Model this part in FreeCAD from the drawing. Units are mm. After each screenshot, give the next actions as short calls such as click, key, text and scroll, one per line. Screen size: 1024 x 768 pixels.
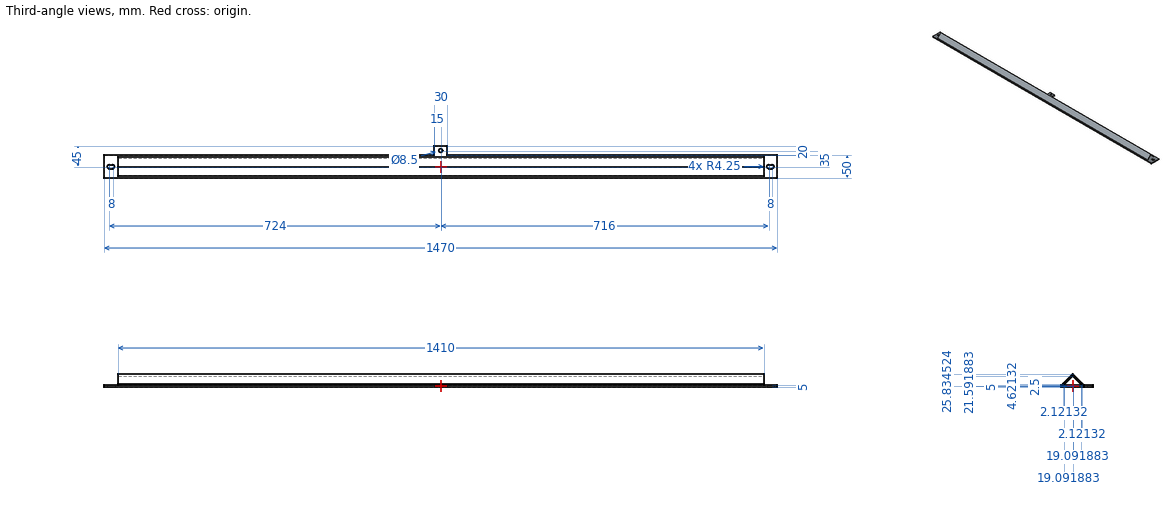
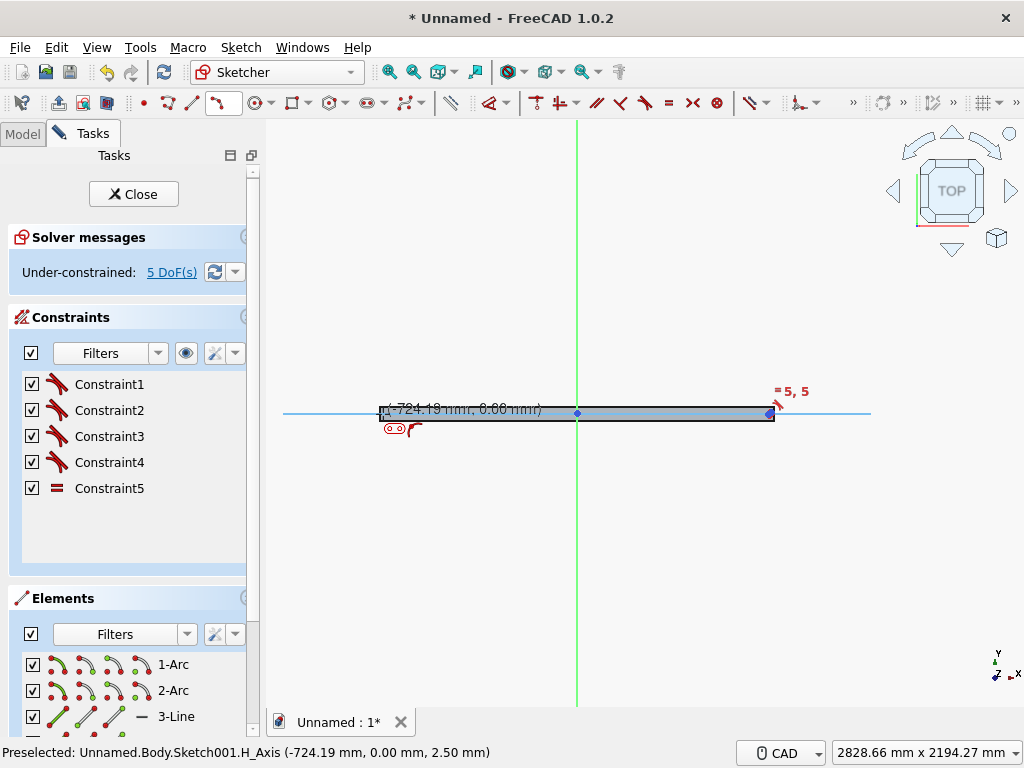
click(383, 414)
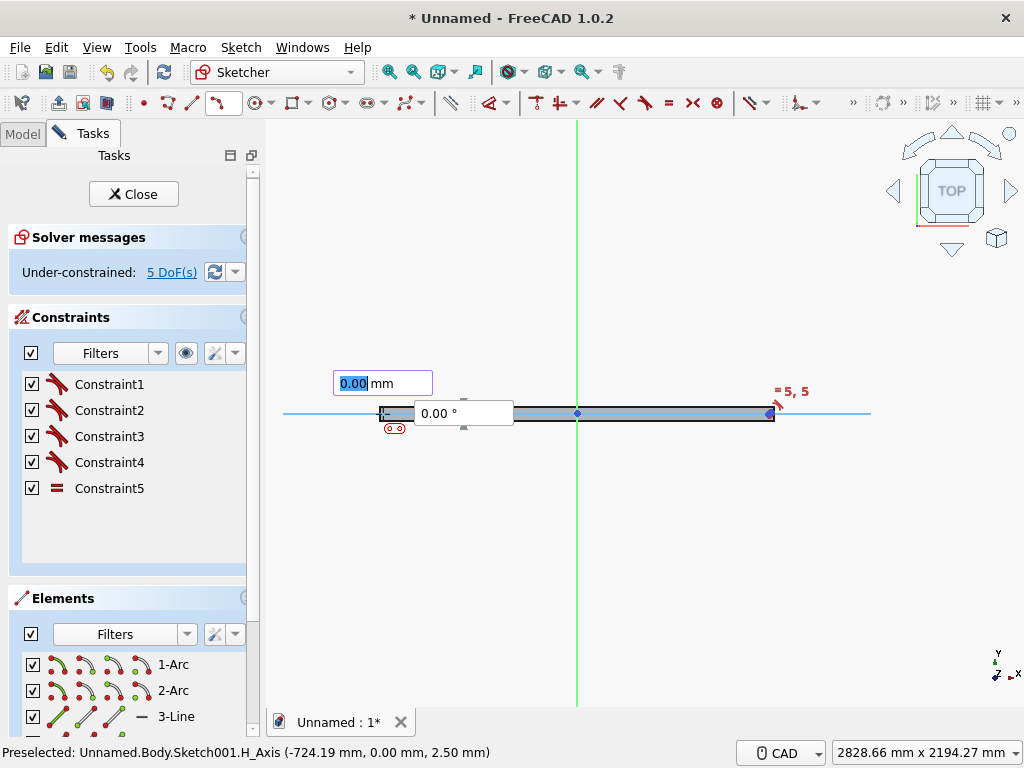
scroll(385, 414, up, 11)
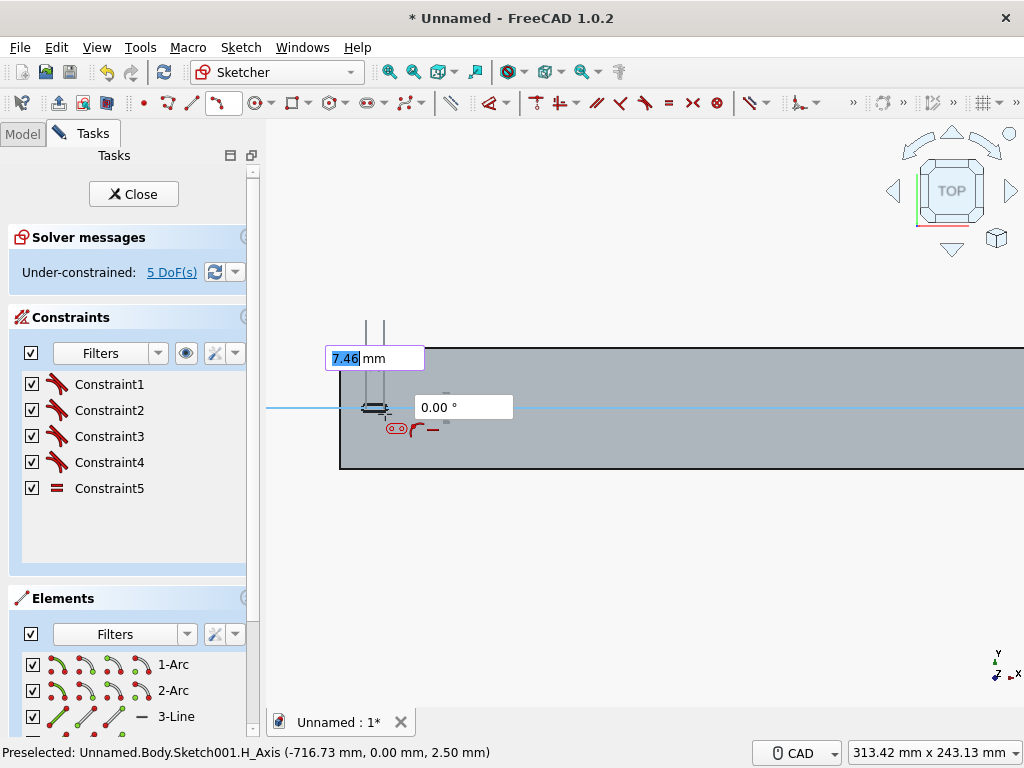
click(386, 399)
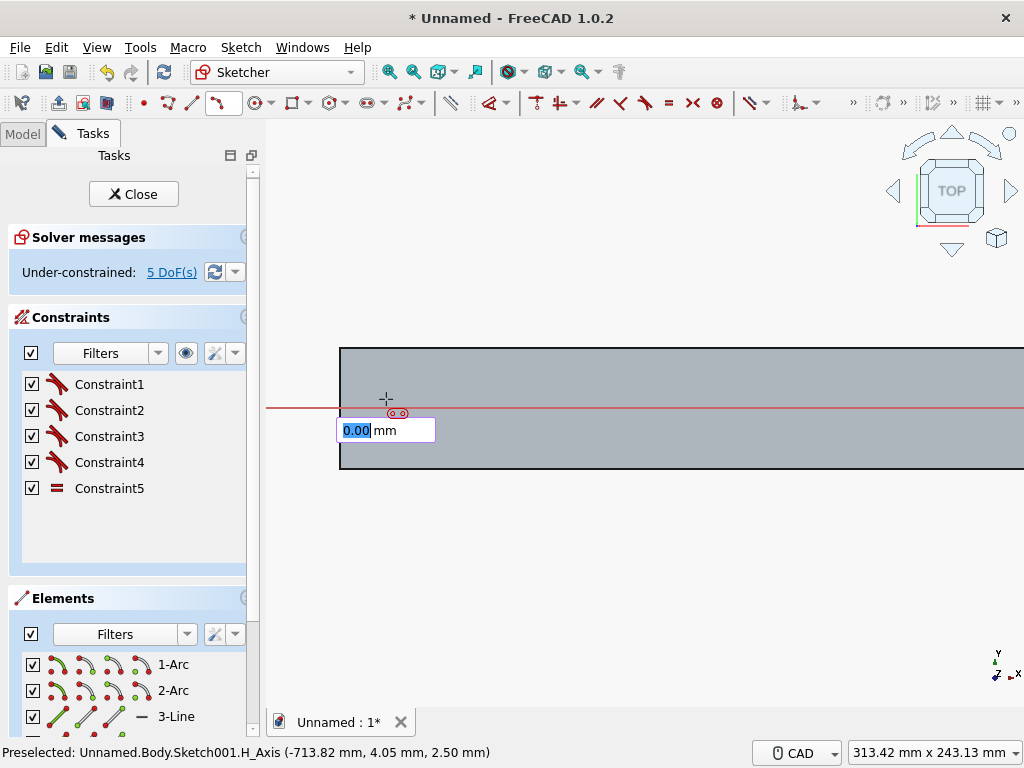
scroll(376, 419, up, 3)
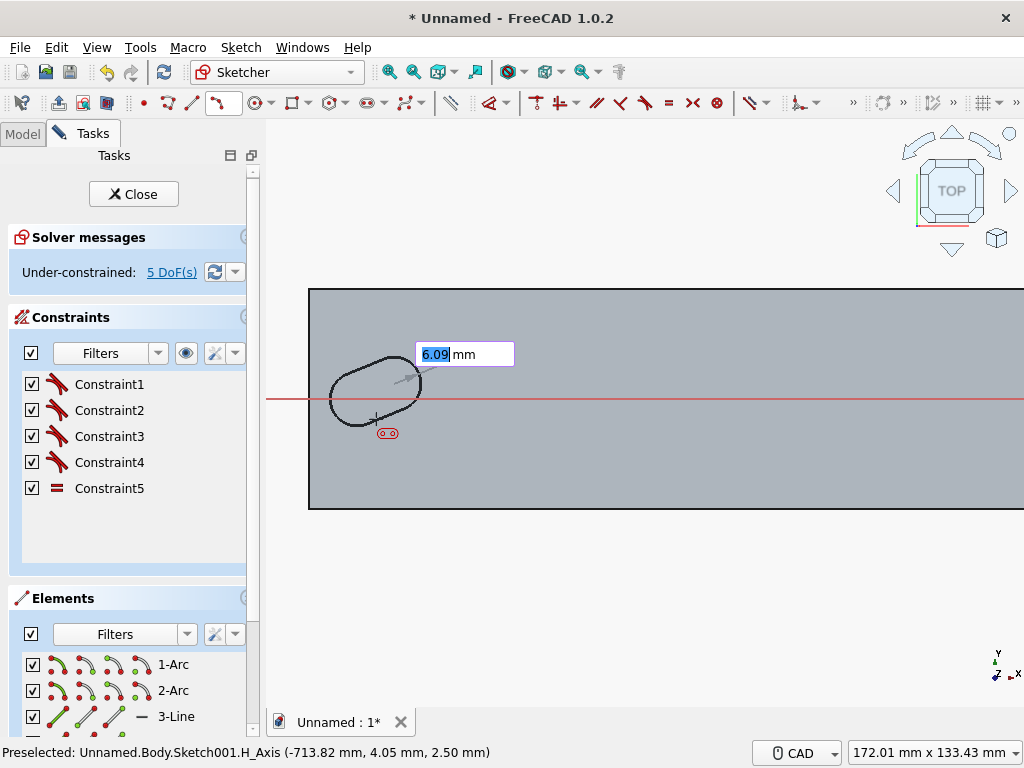
click(376, 418)
key(Escape)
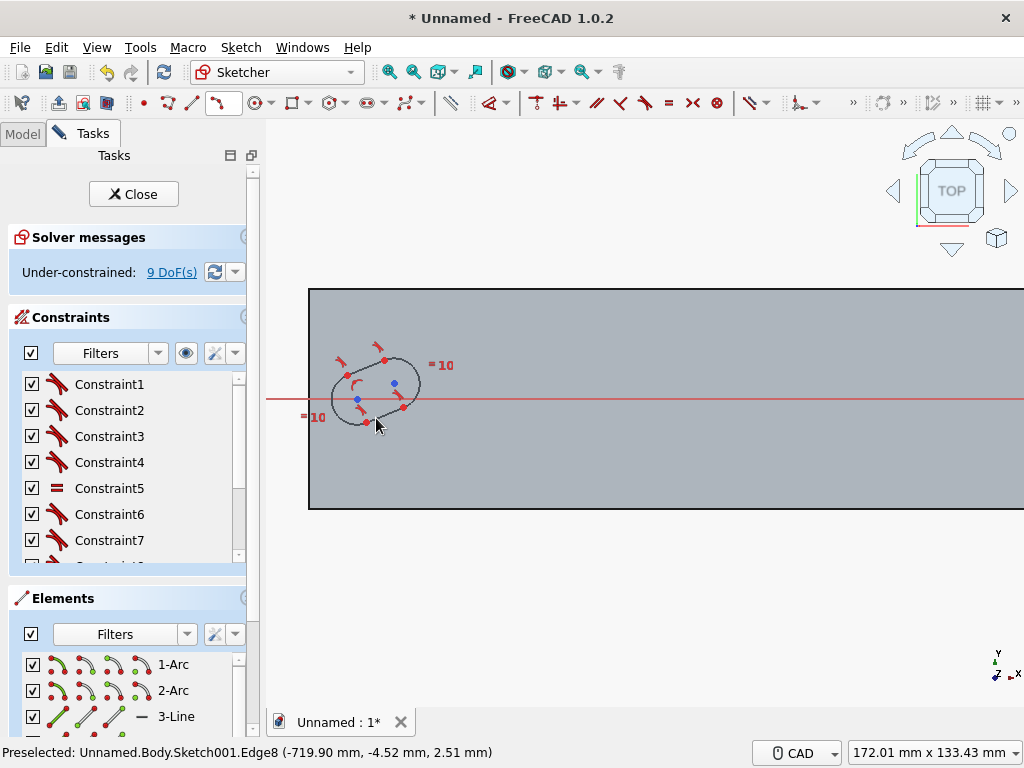
scroll(384, 414, down, 14)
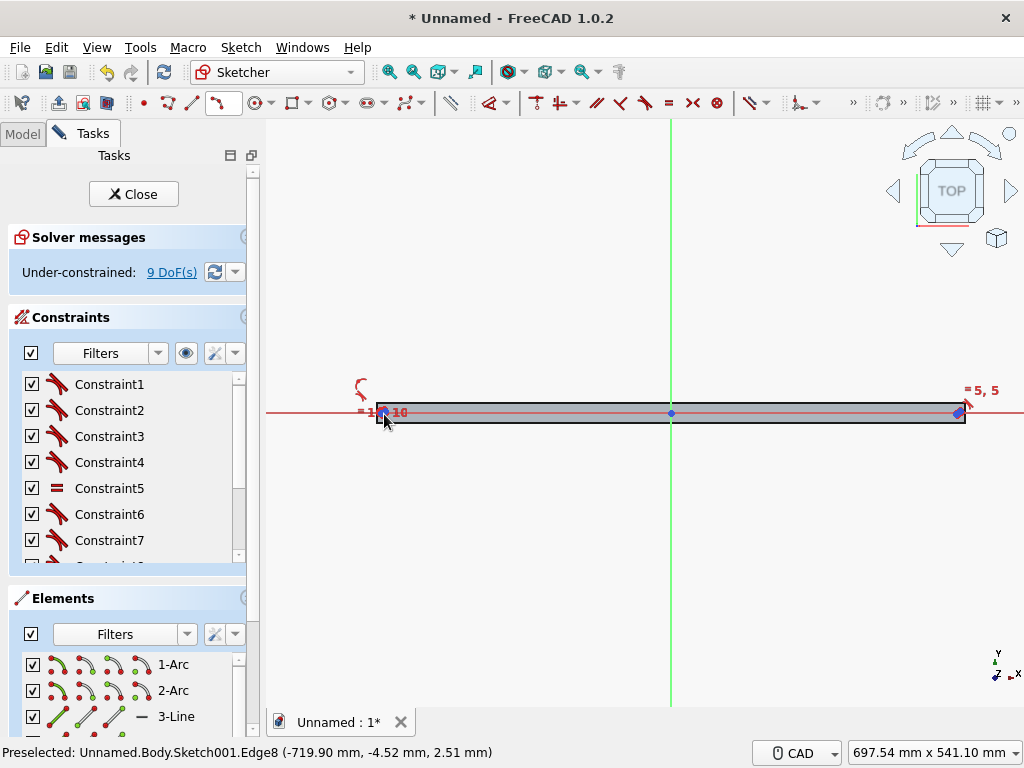
scroll(769, 413, up, 14)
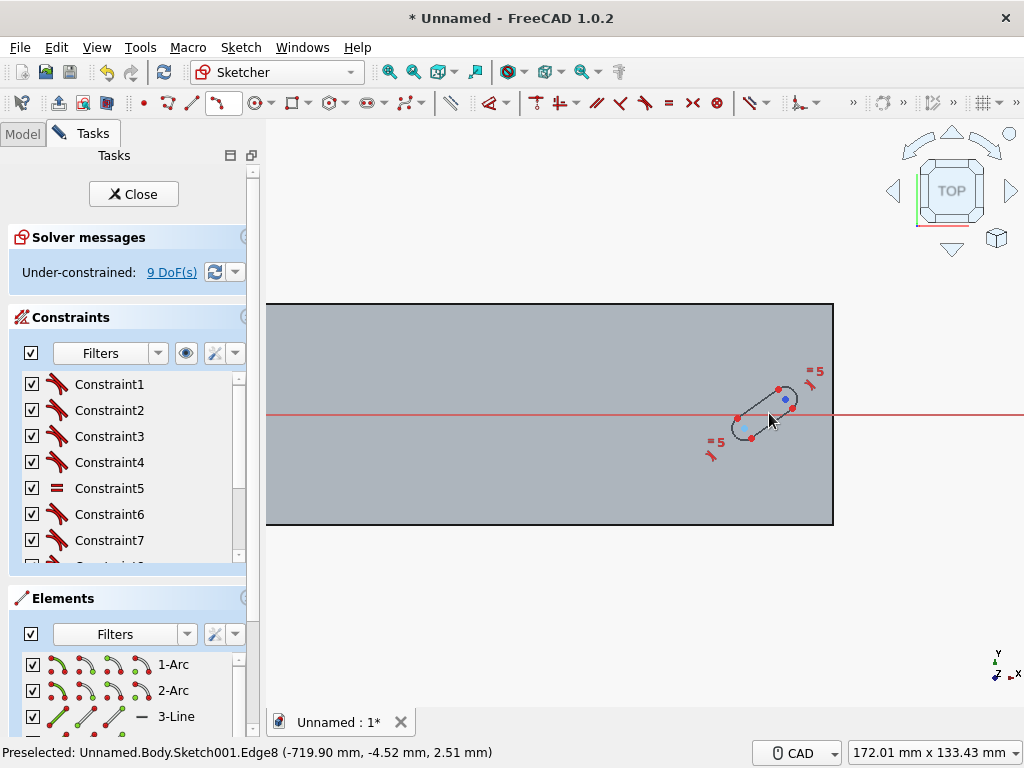
click(766, 398)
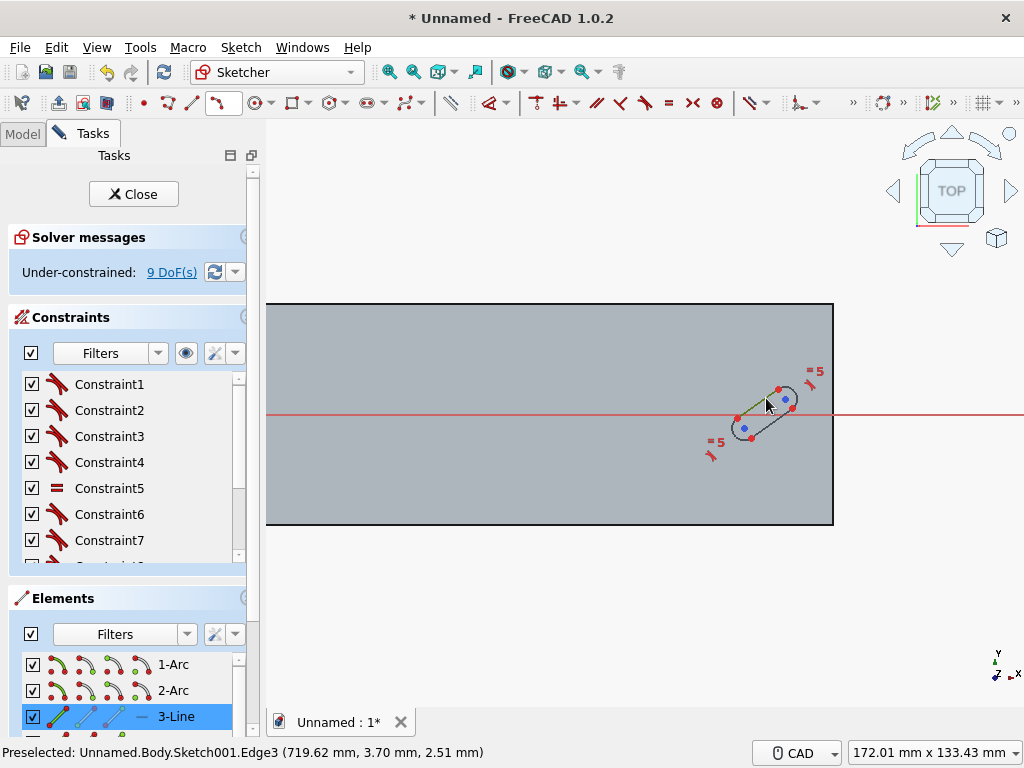
click(578, 104)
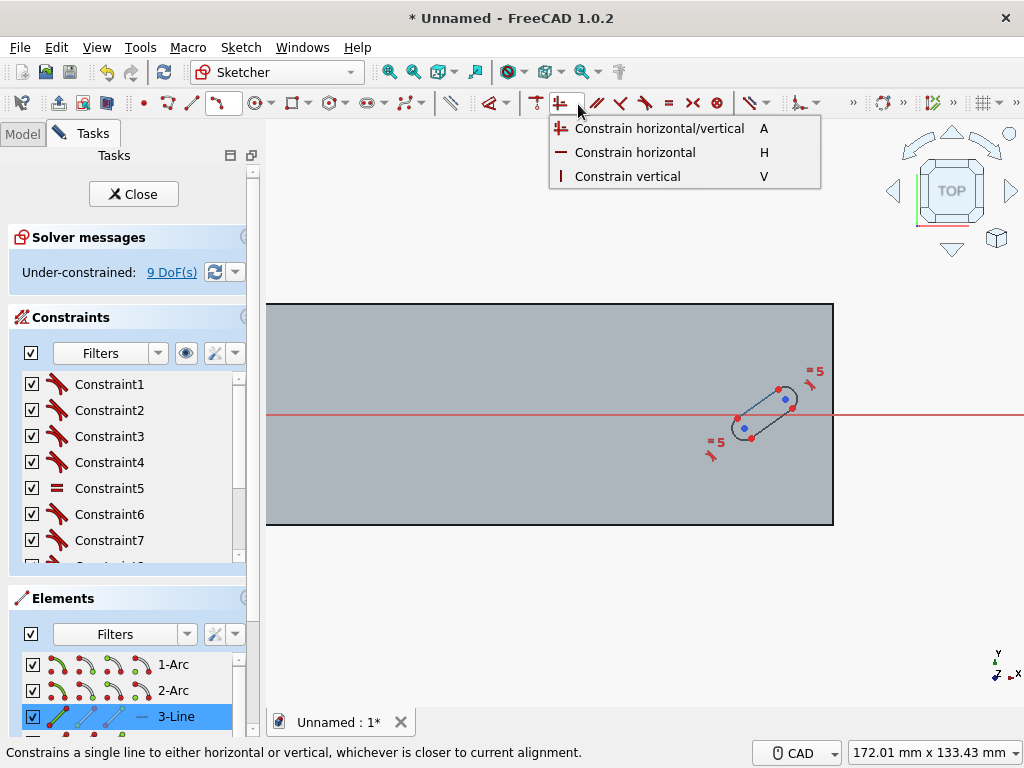
click(685, 152)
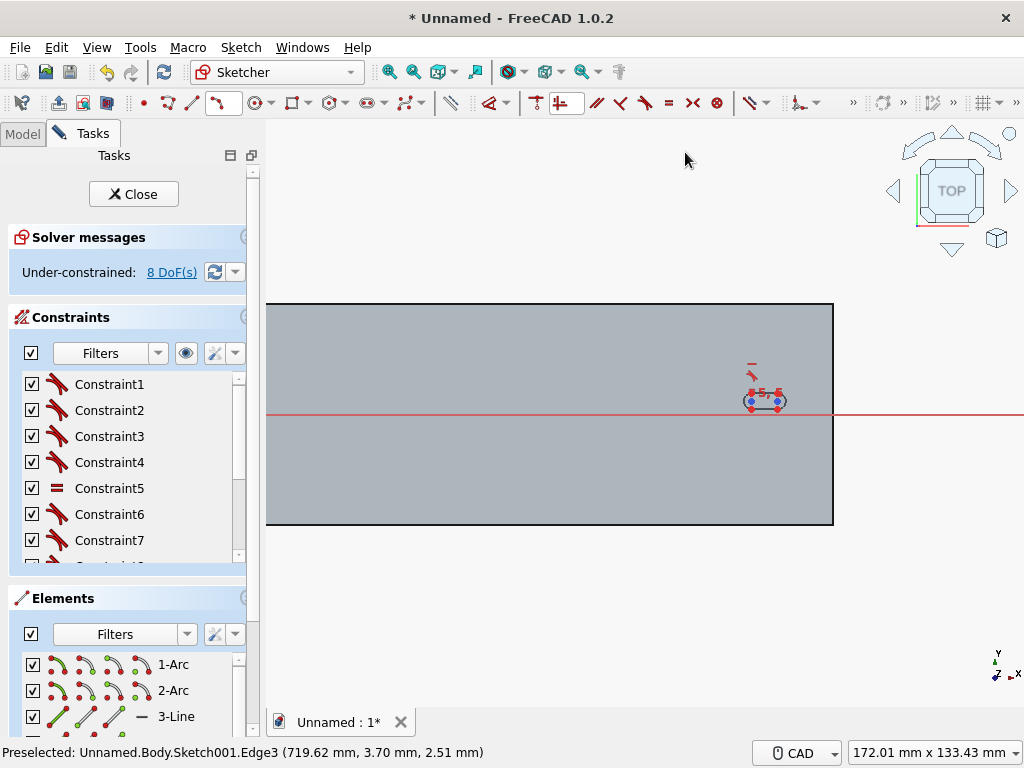
scroll(770, 413, down, 14)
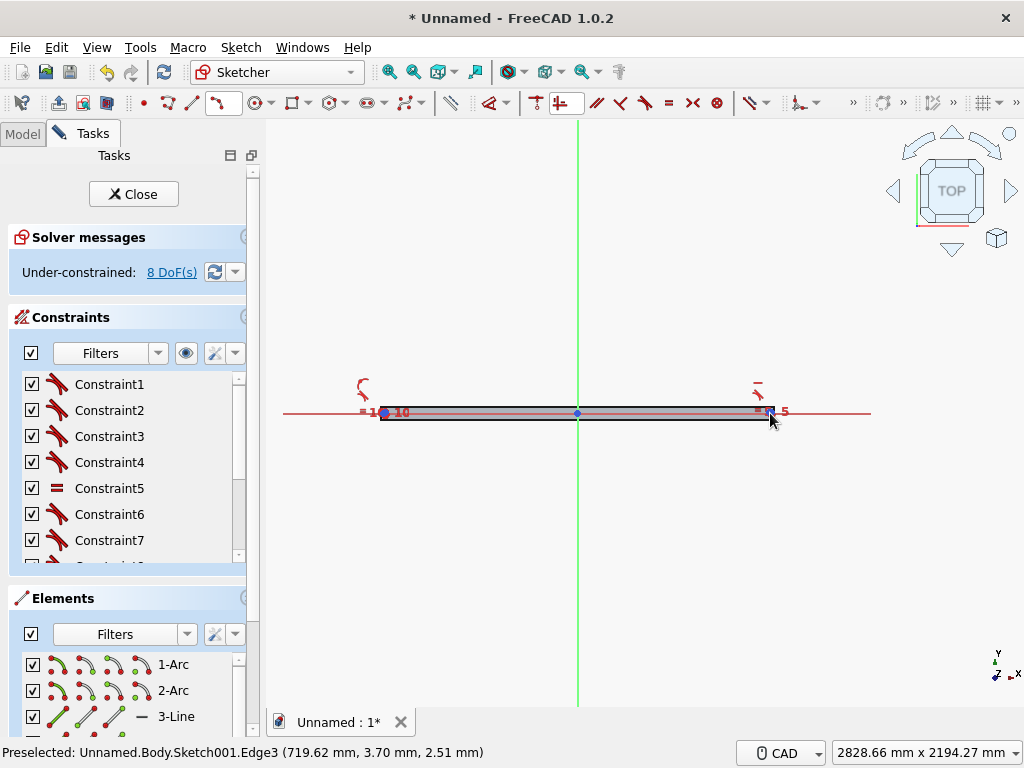
scroll(384, 412, up, 14)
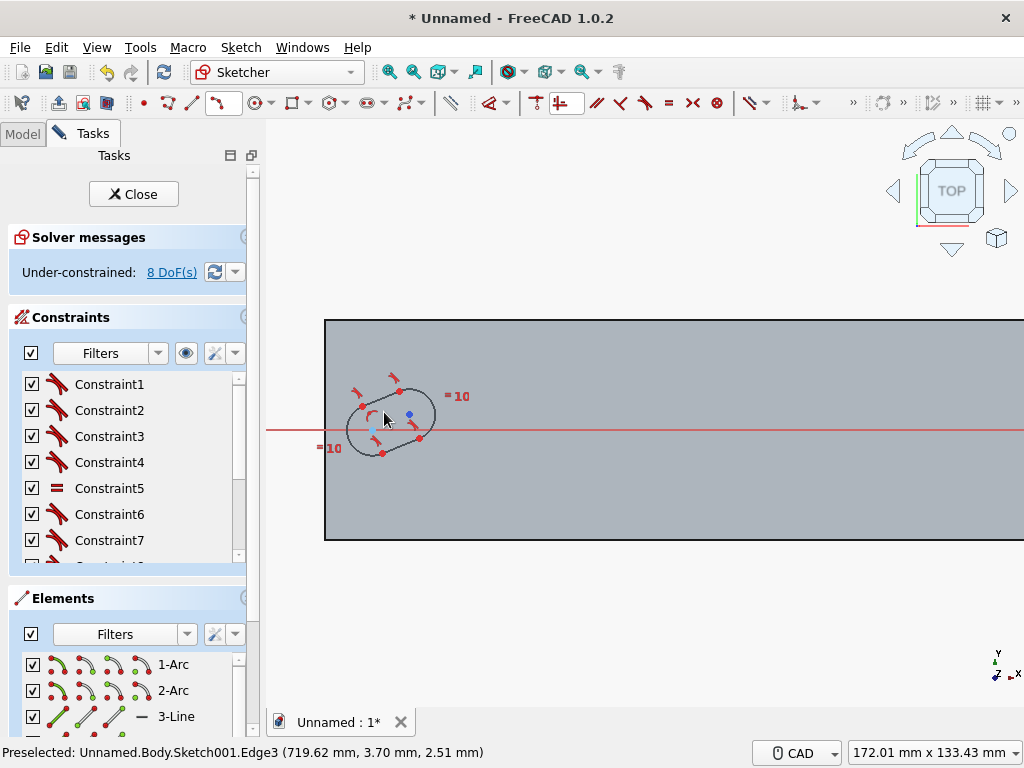
click(374, 402)